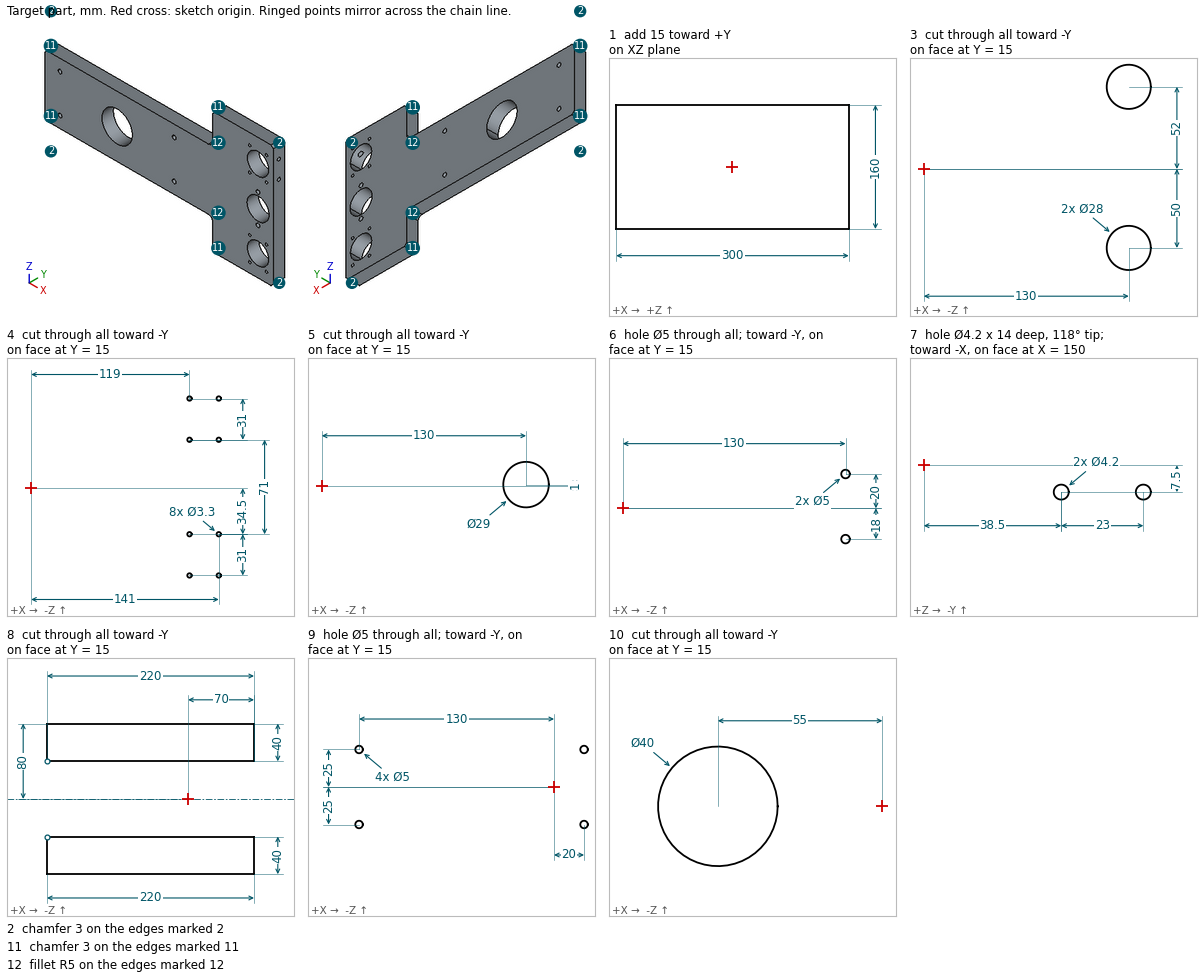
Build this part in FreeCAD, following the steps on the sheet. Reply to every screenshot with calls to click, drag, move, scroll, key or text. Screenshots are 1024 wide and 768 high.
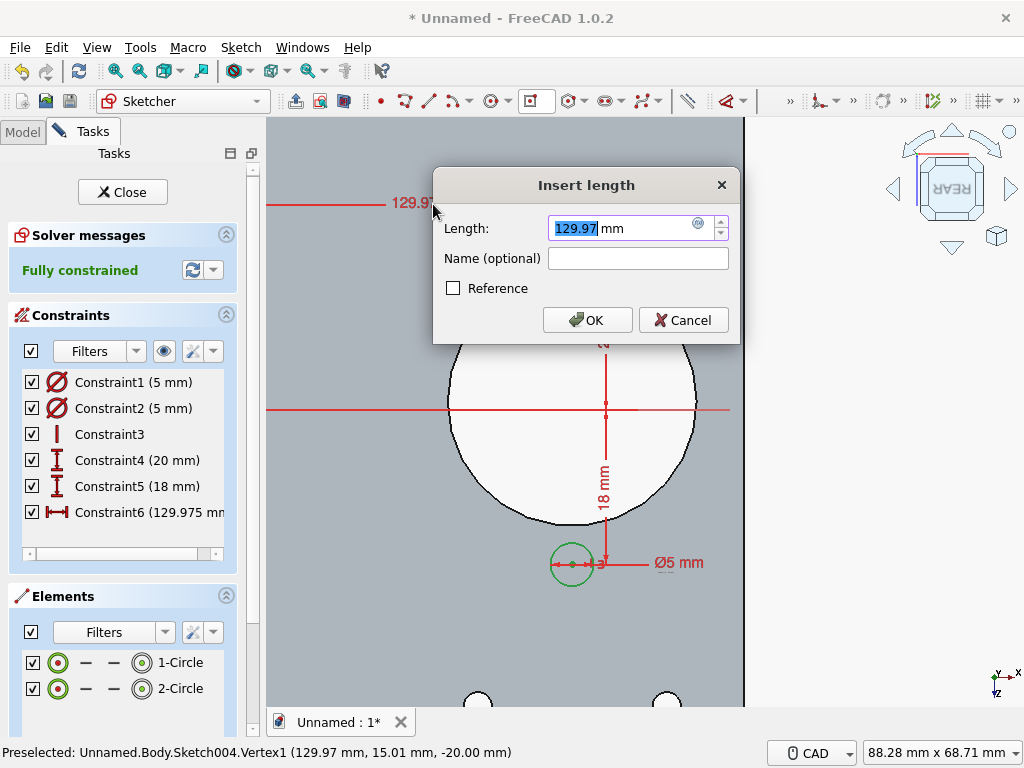
text(130)
key(Return)
key(Escape)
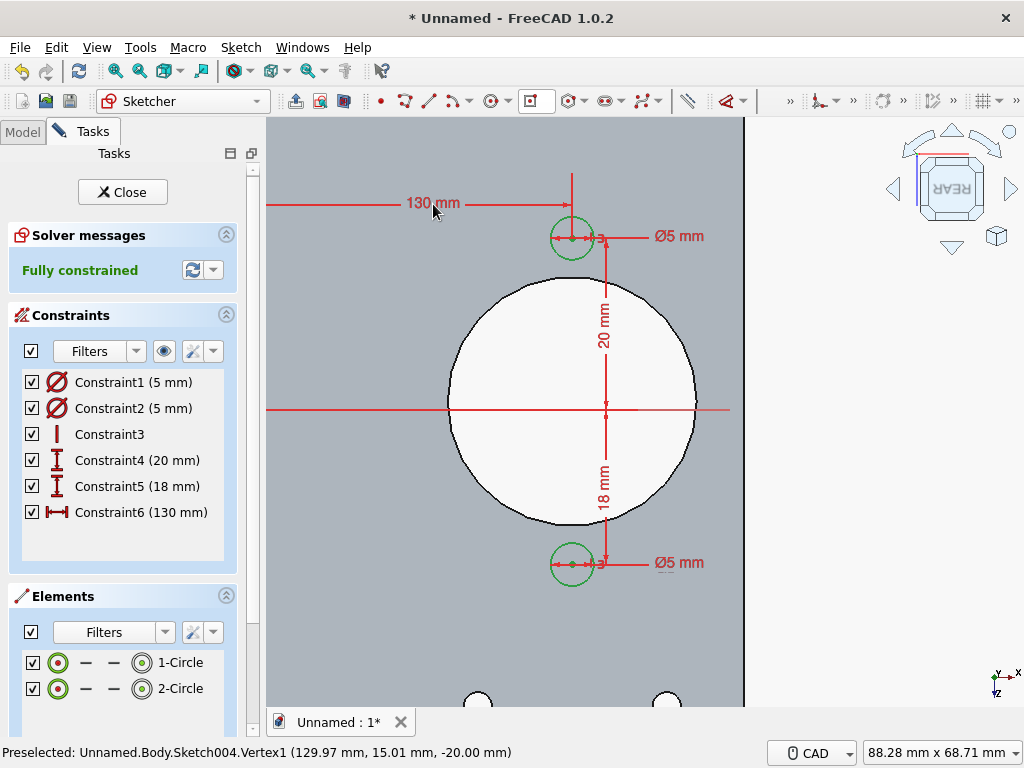
click(123, 192)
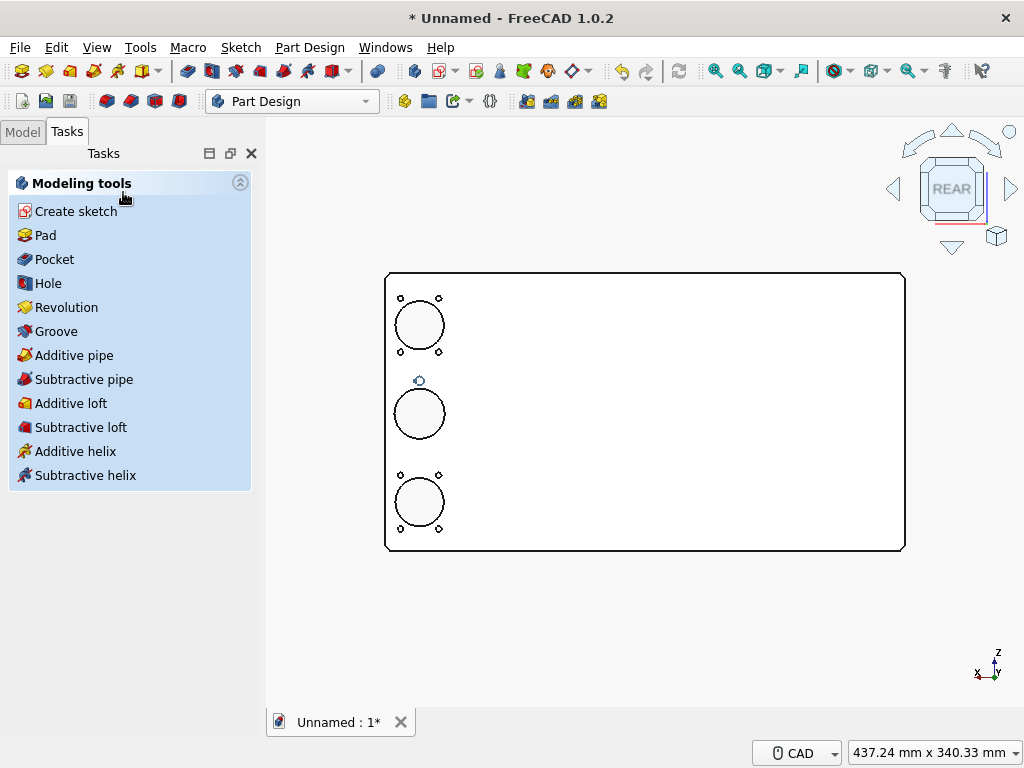
click(212, 72)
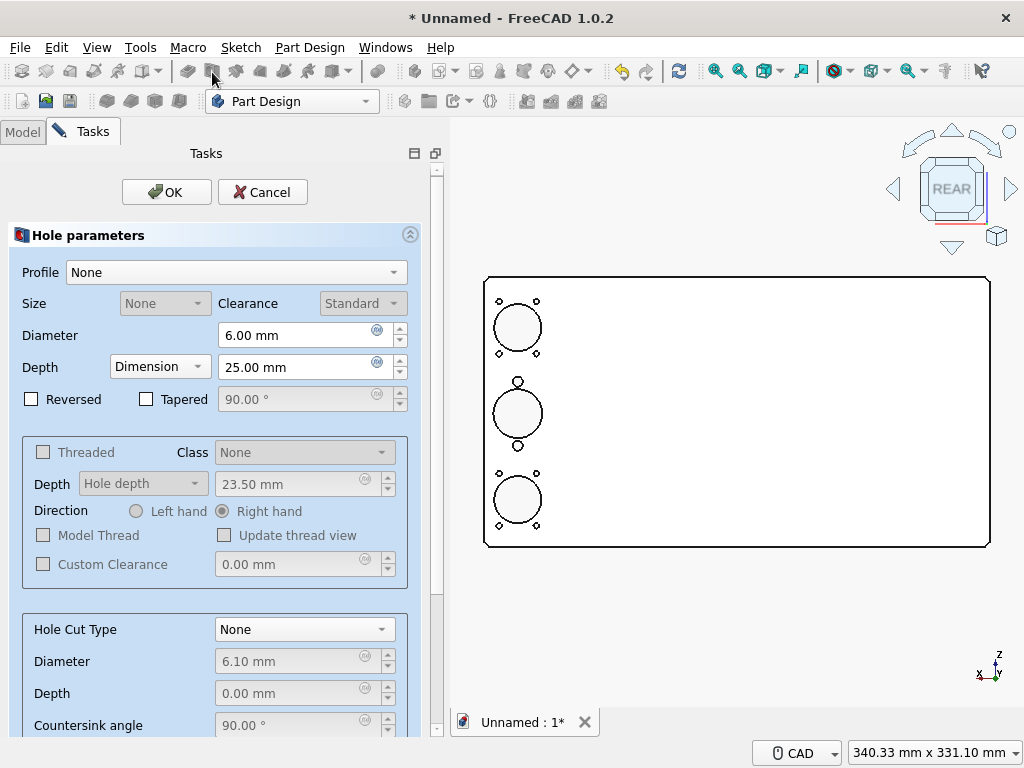
triple_click(305, 335)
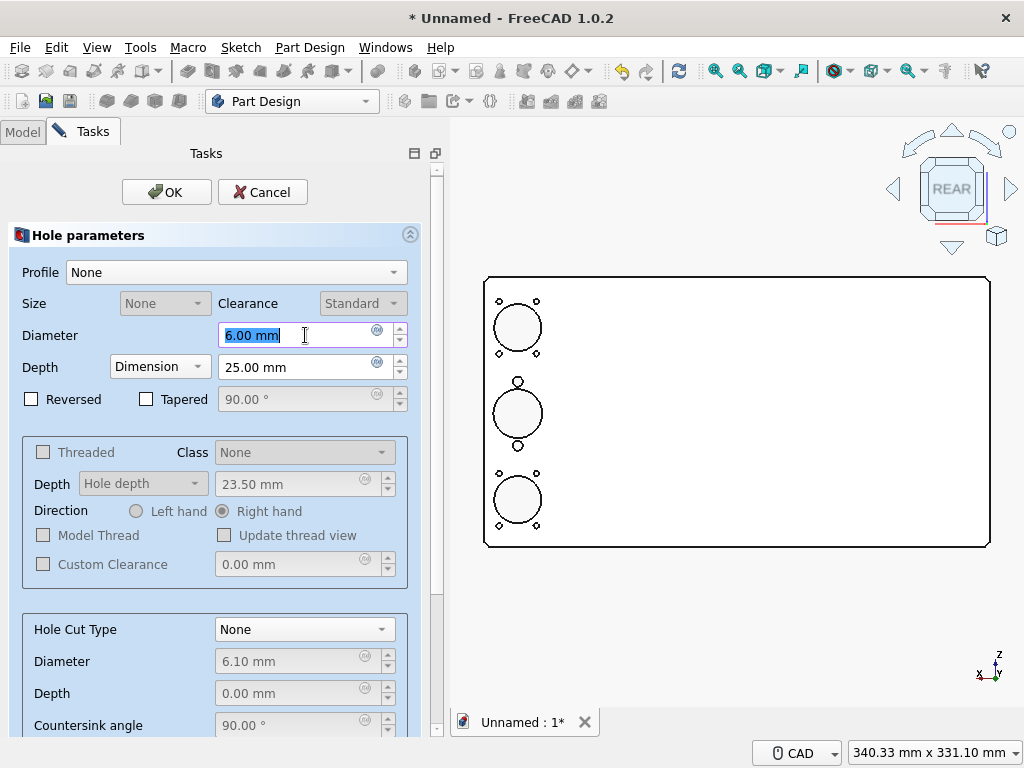
text(5)
key(Tab)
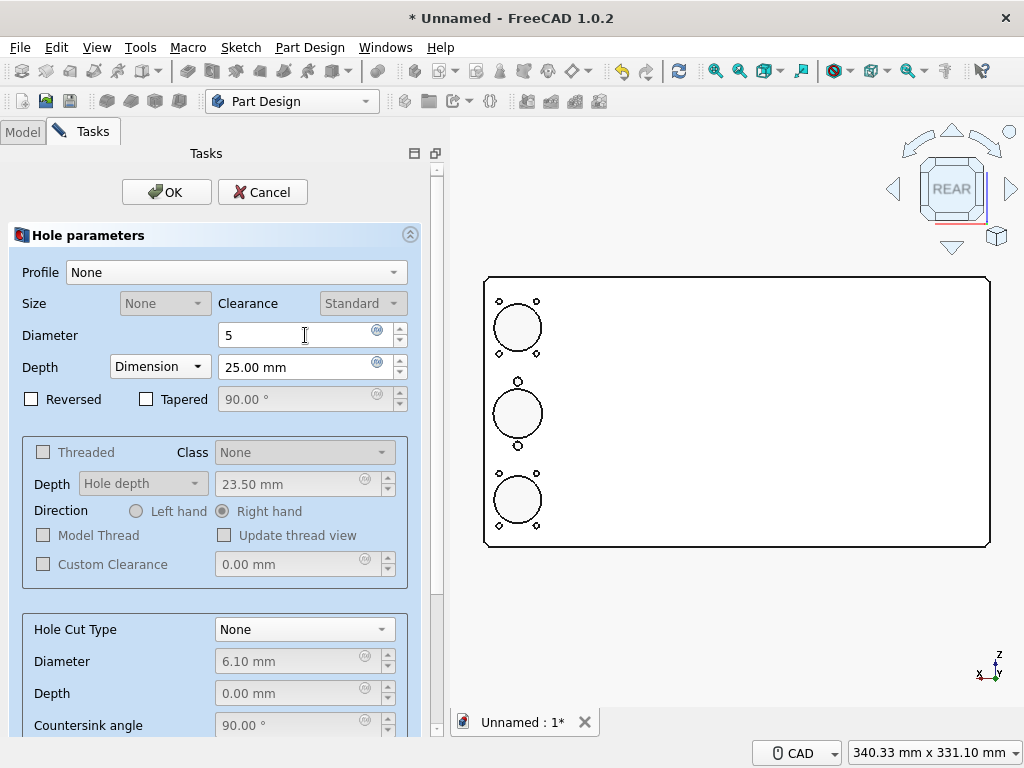
click(161, 366)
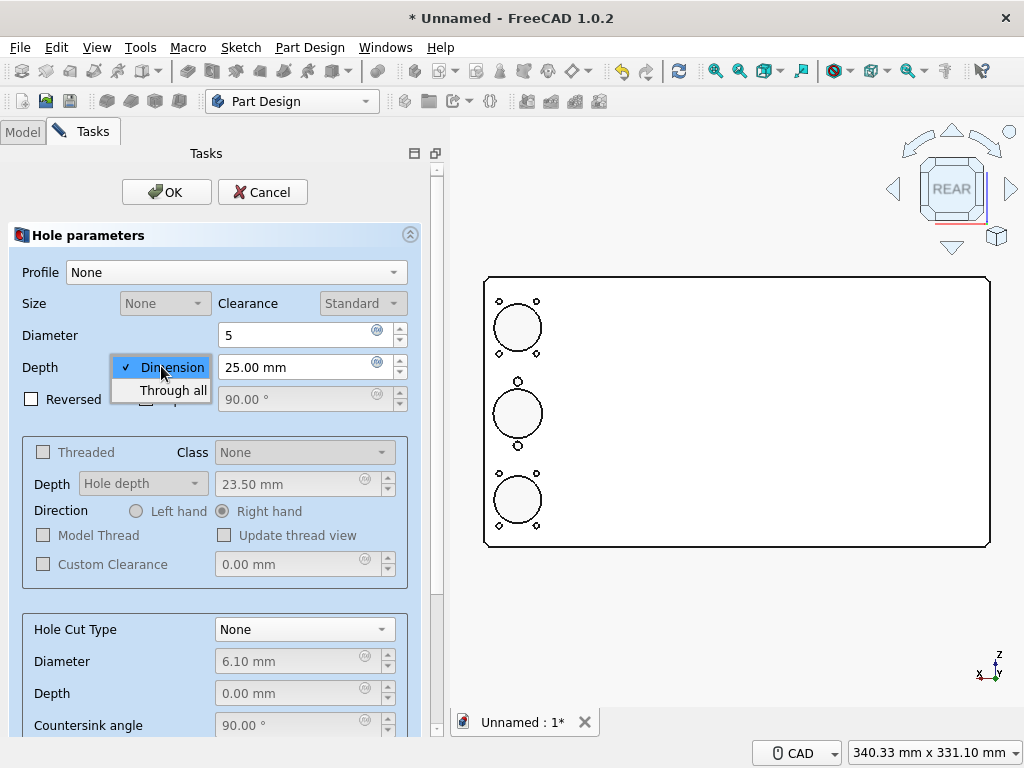
click(160, 390)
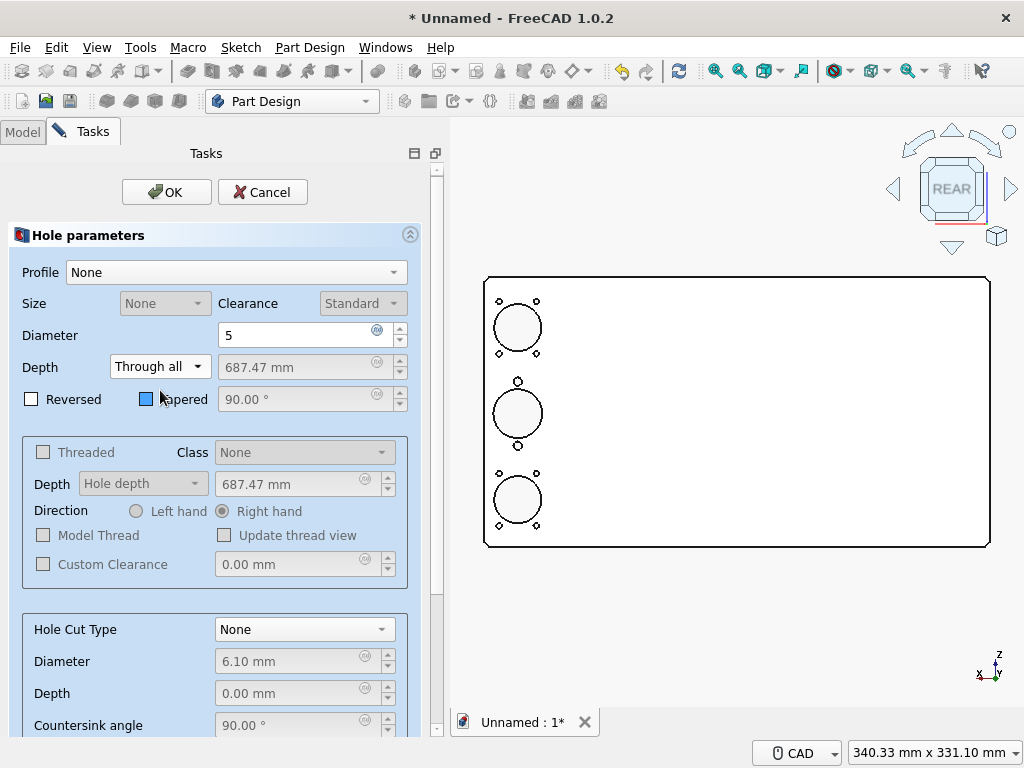
click(167, 192)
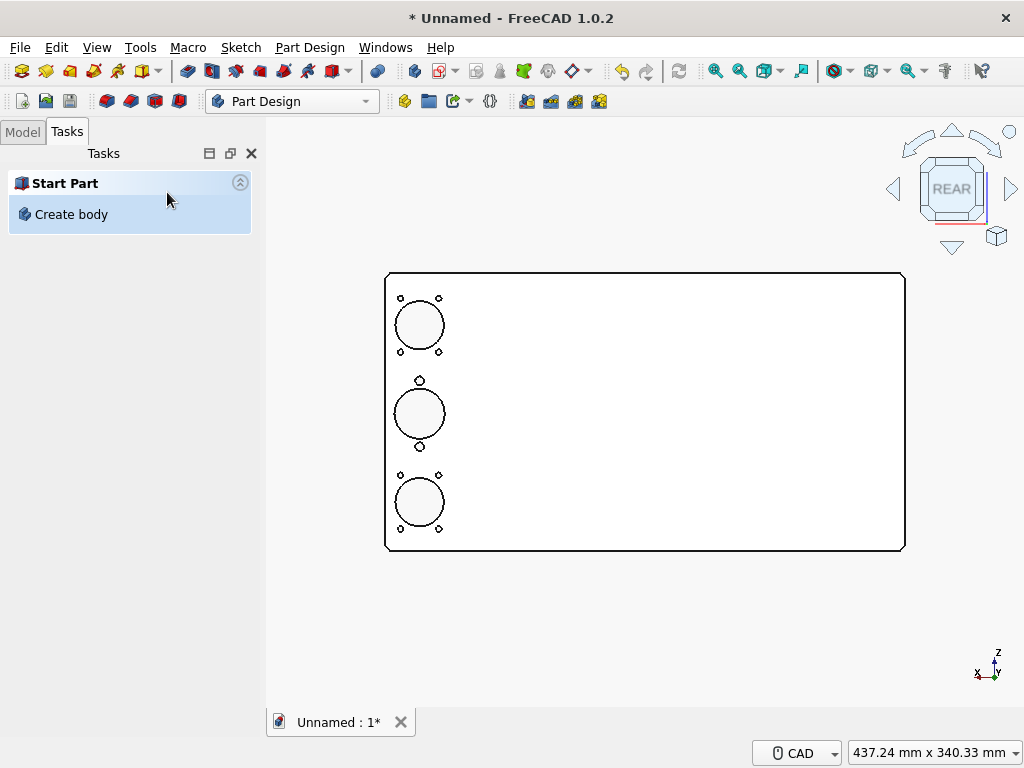
key(0)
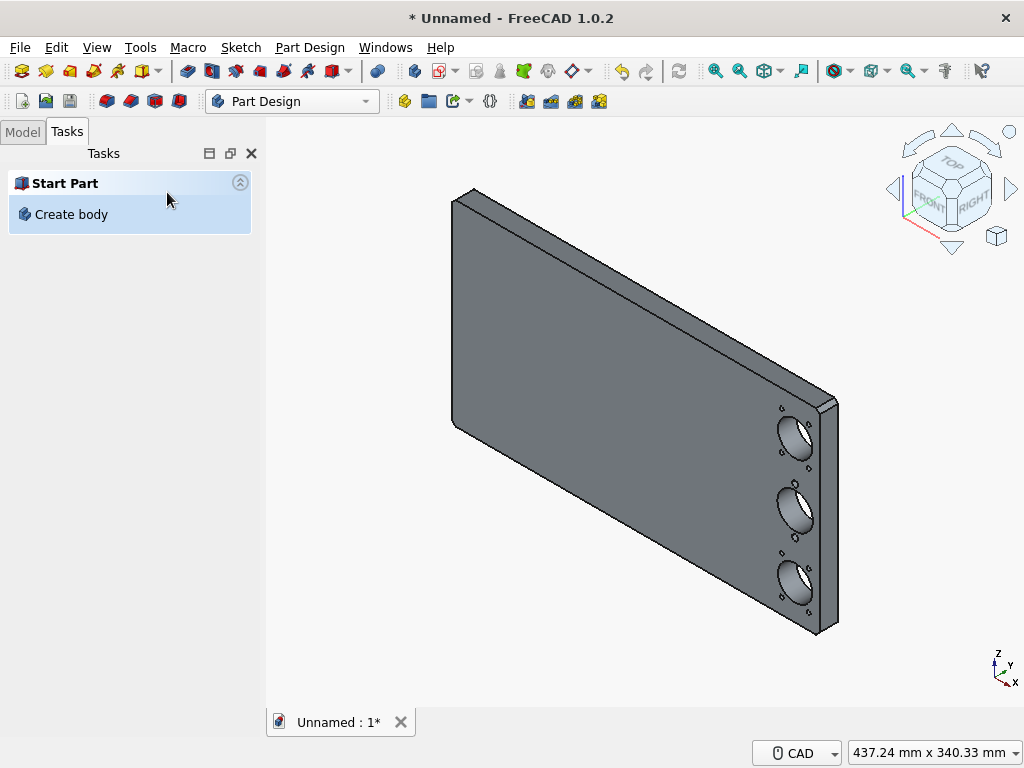
click(829, 424)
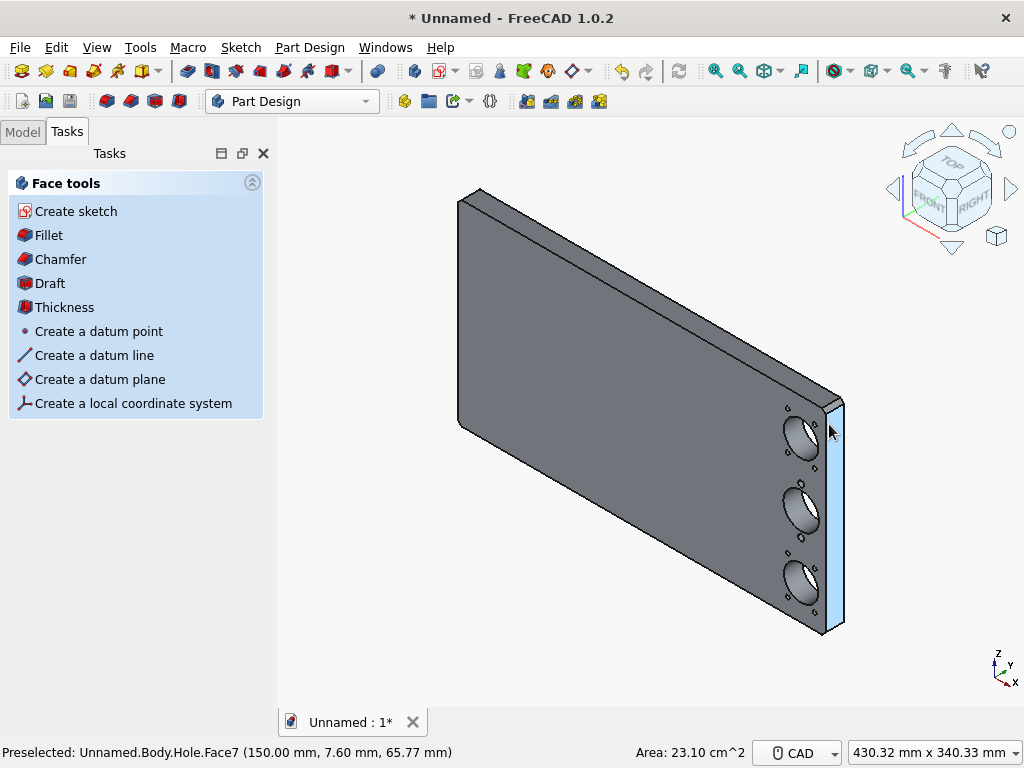
click(440, 72)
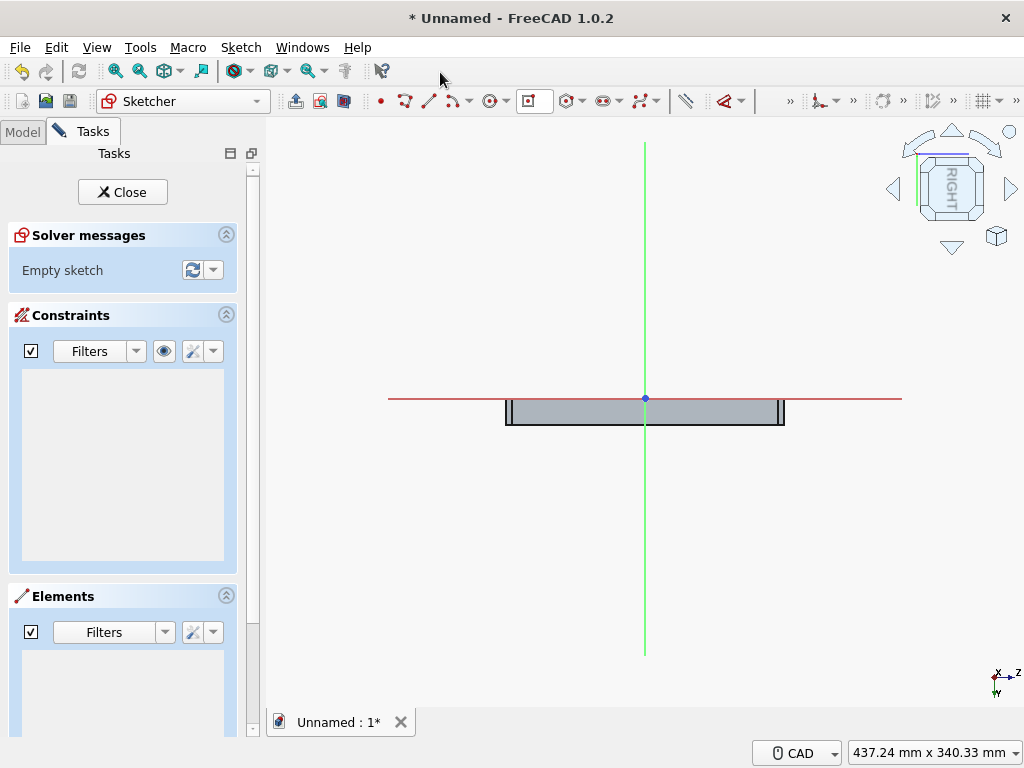
scroll(753, 405, up, 6)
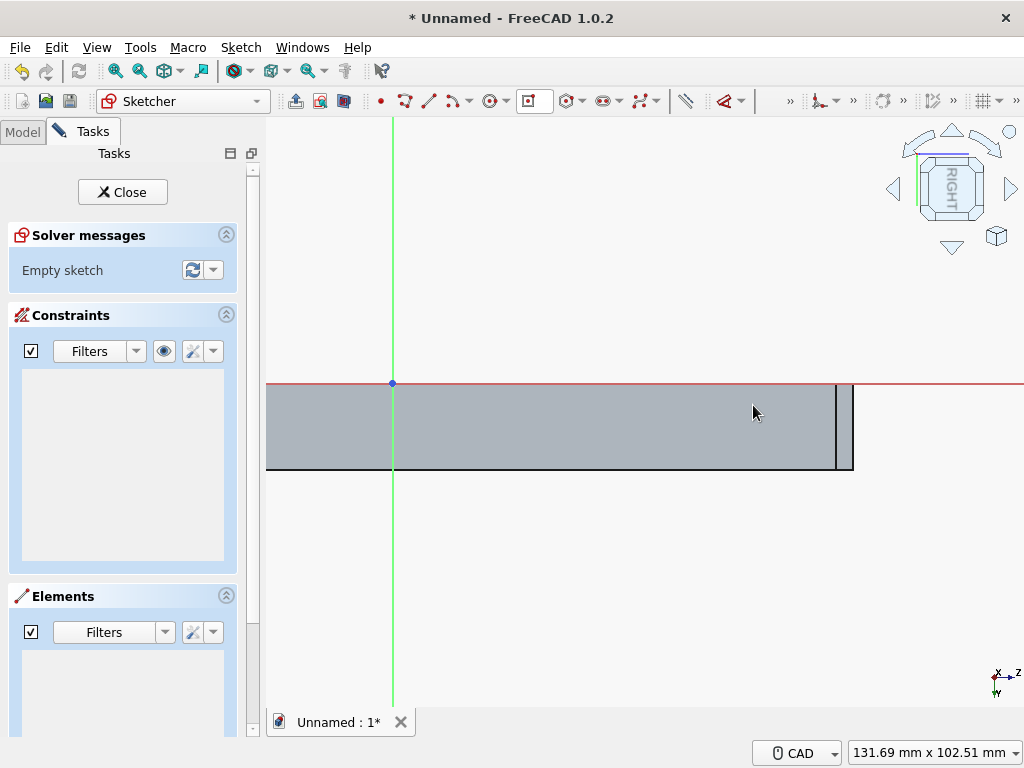
click(490, 102)